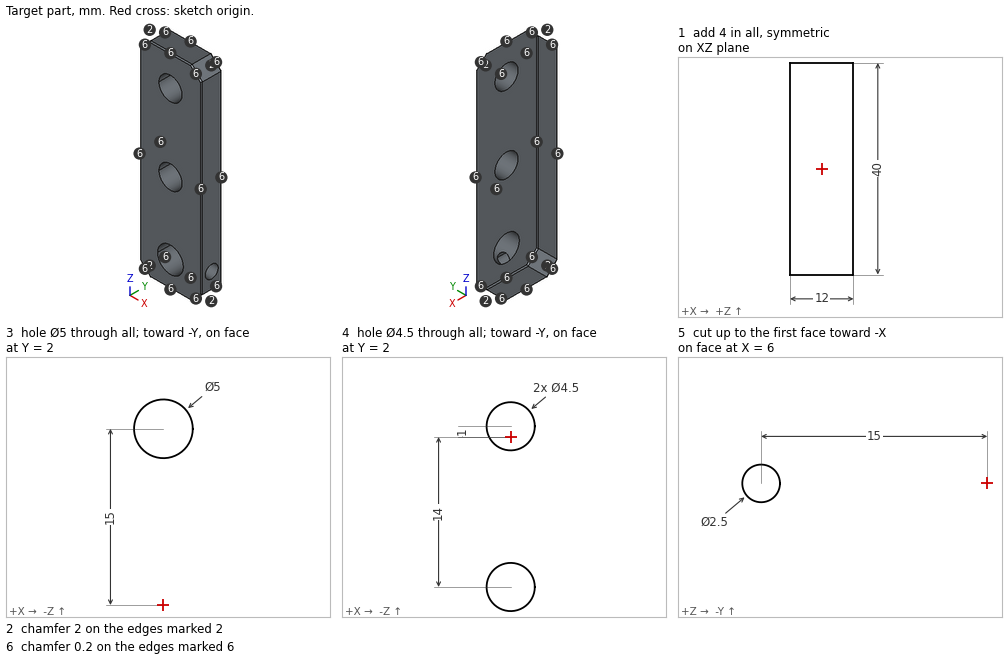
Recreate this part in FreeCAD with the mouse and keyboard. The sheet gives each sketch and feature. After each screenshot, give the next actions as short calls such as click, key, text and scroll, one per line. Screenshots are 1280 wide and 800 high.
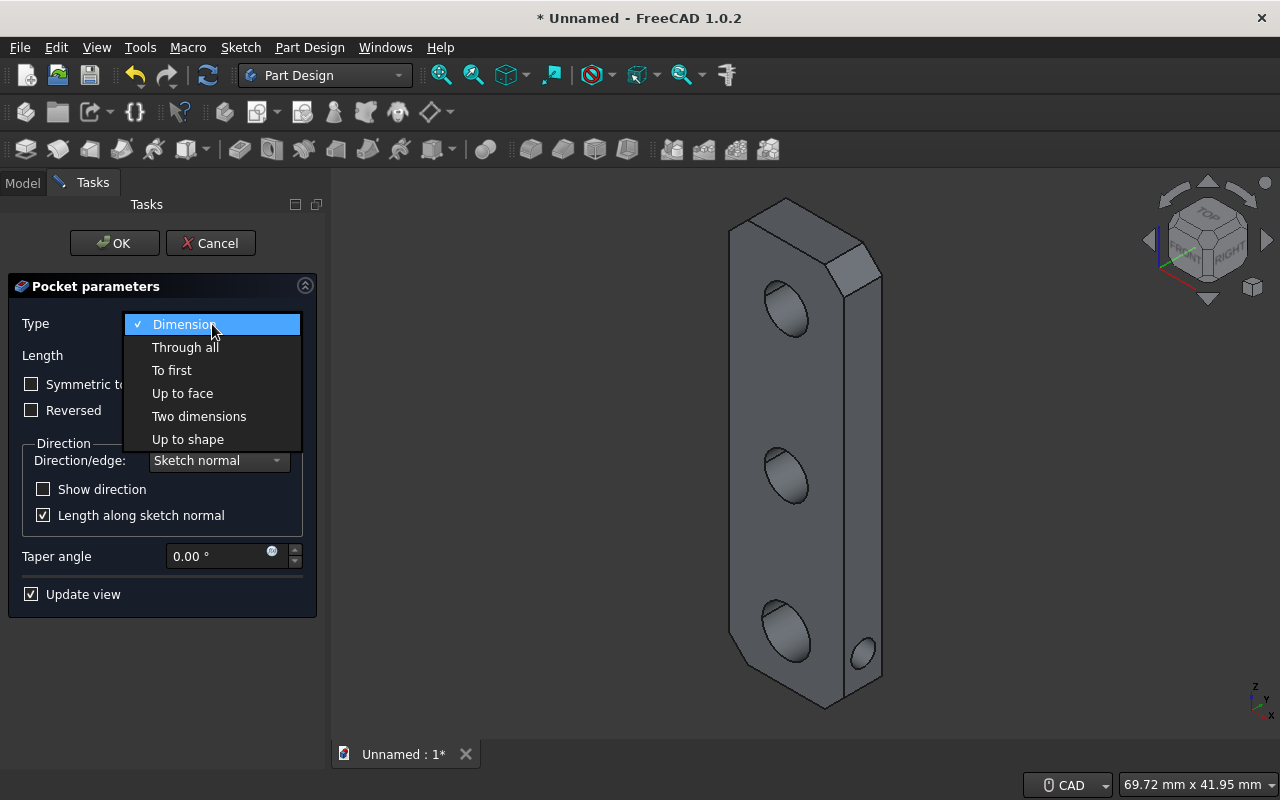
click(212, 370)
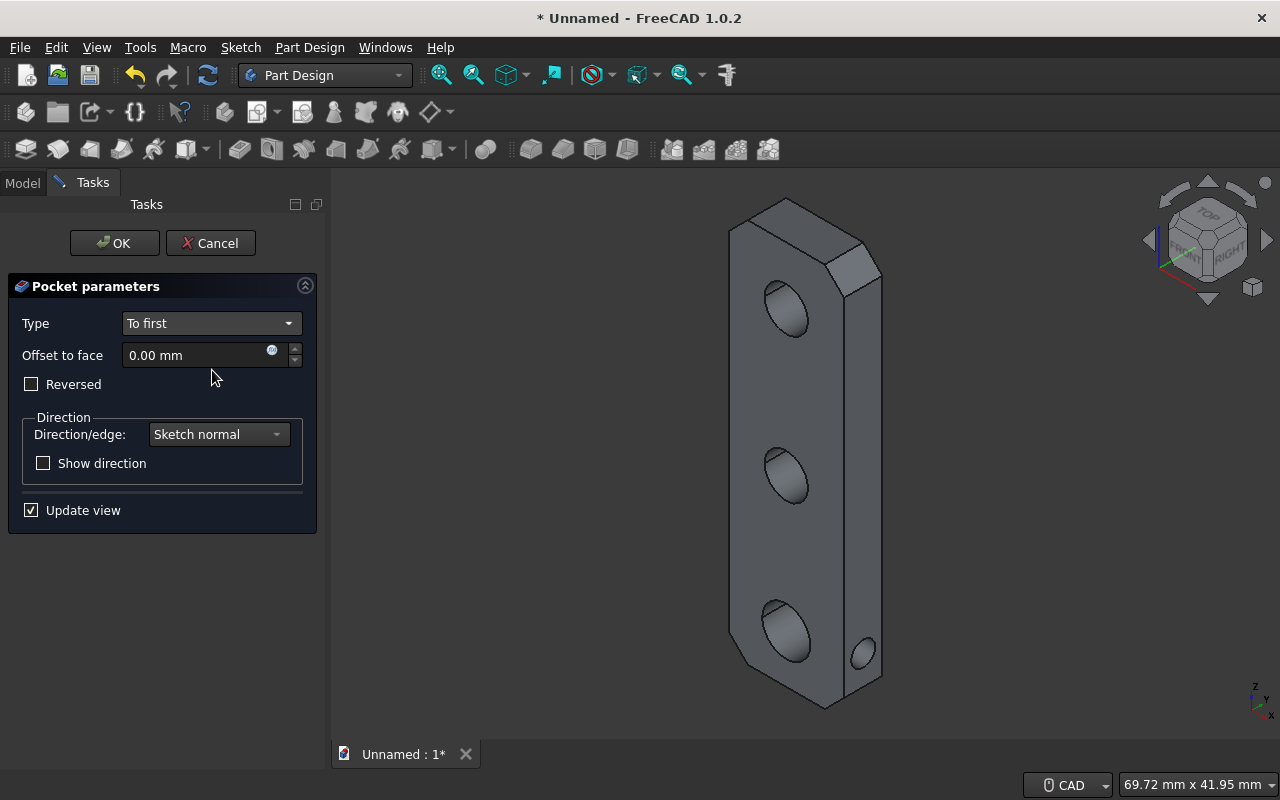
click(115, 243)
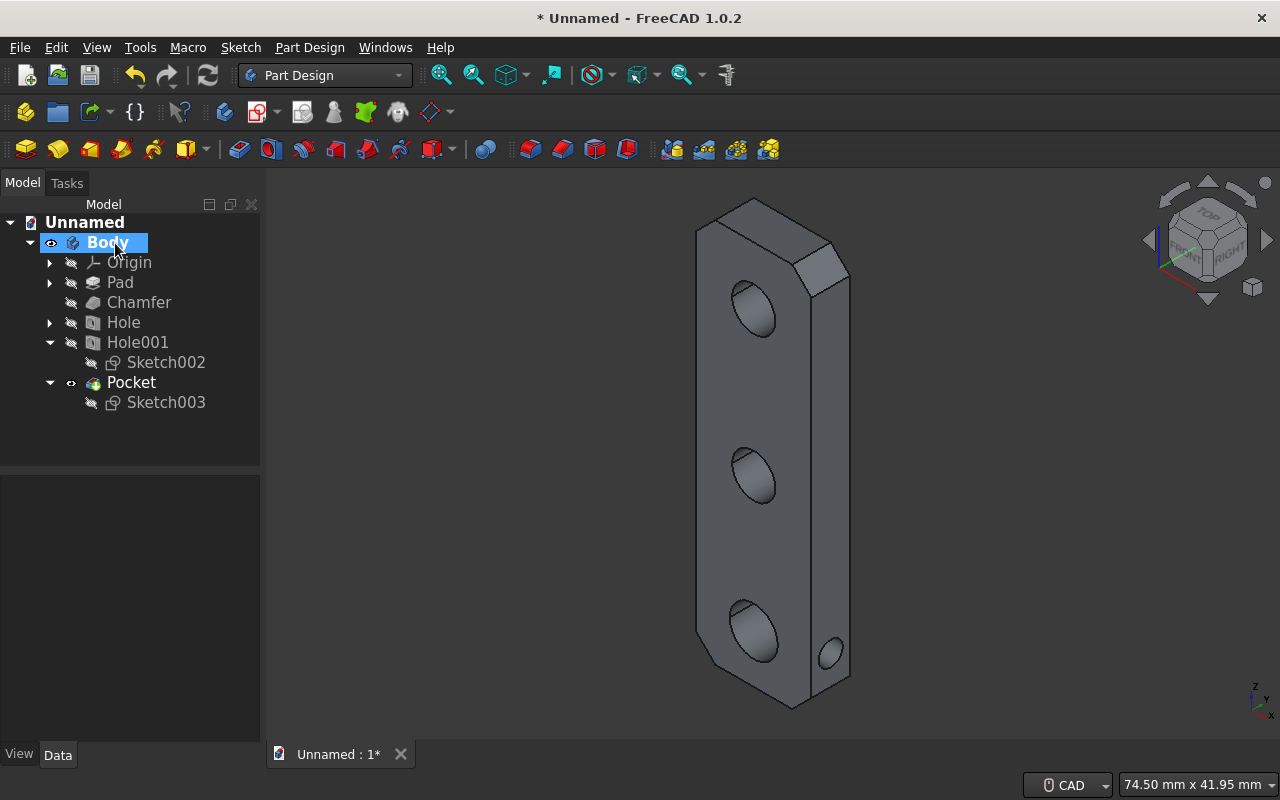
click(811, 497)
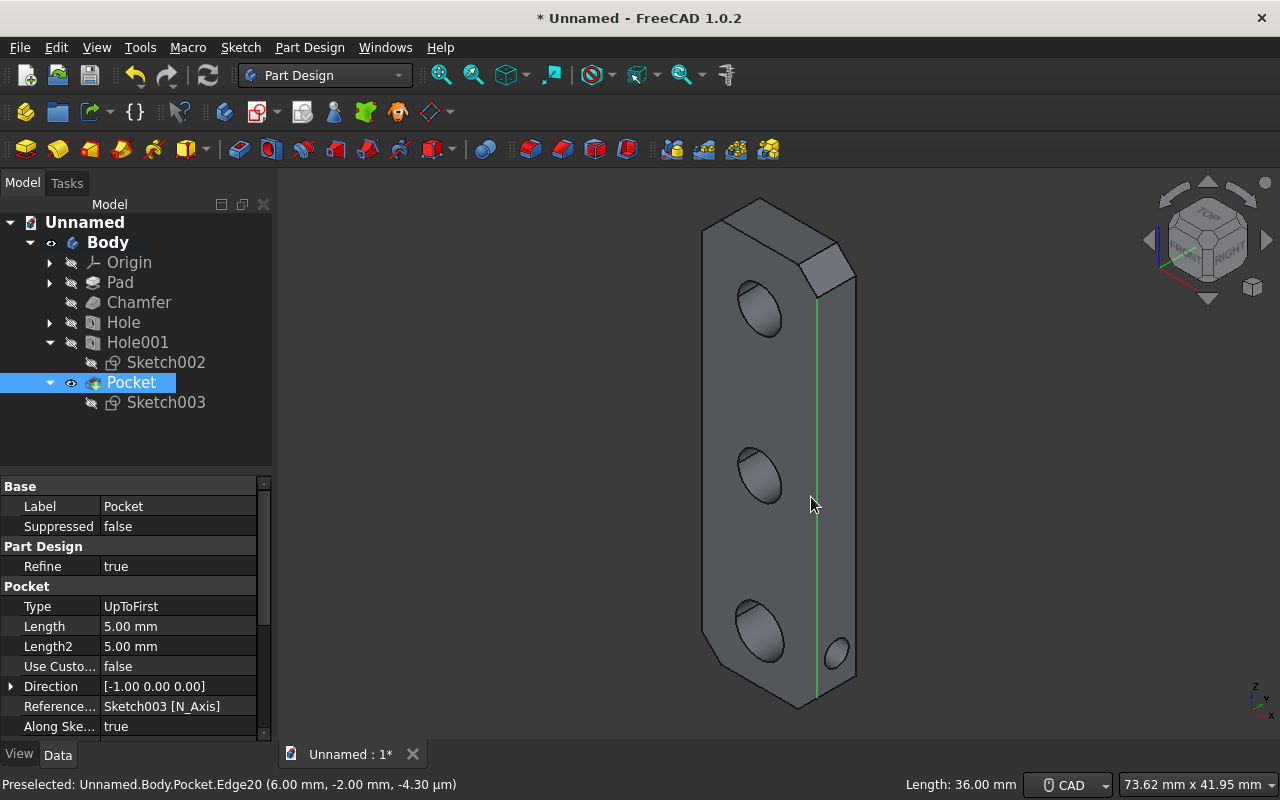
click(760, 241, ctrl)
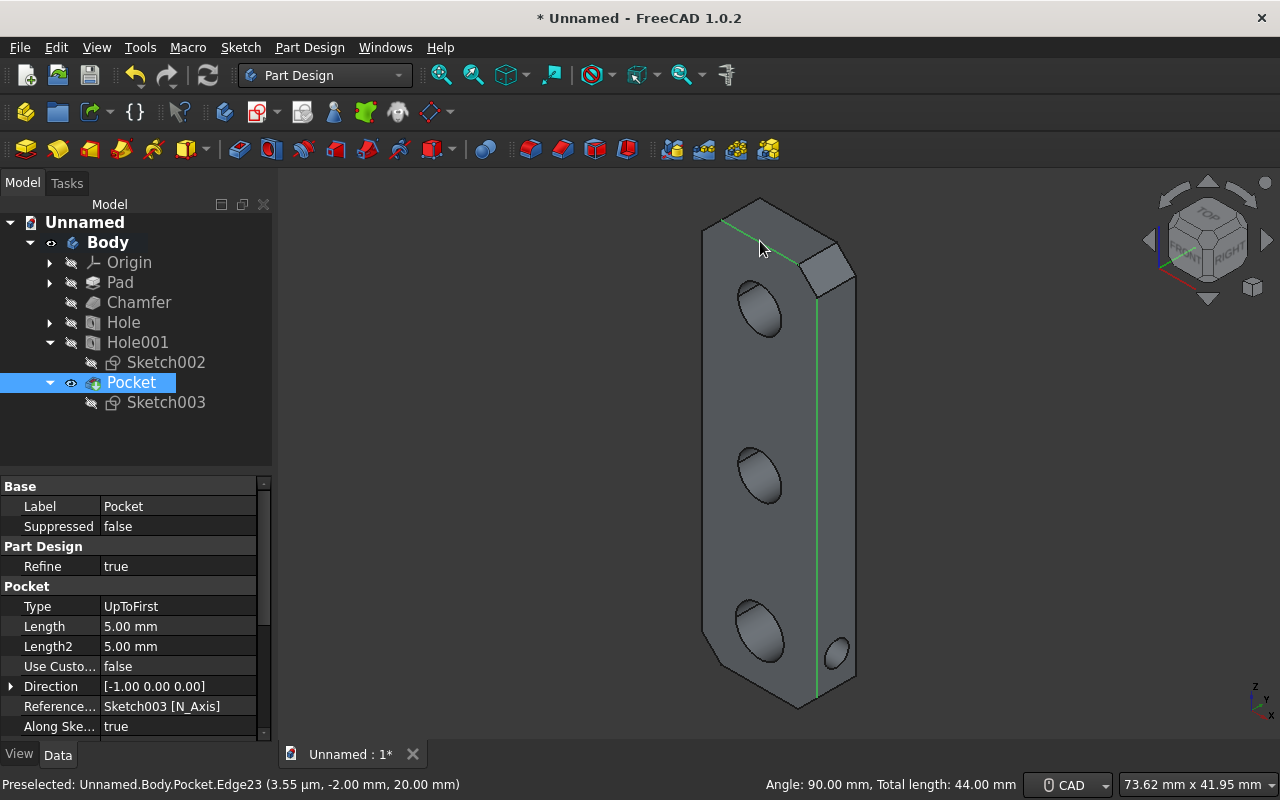
click(712, 225, ctrl)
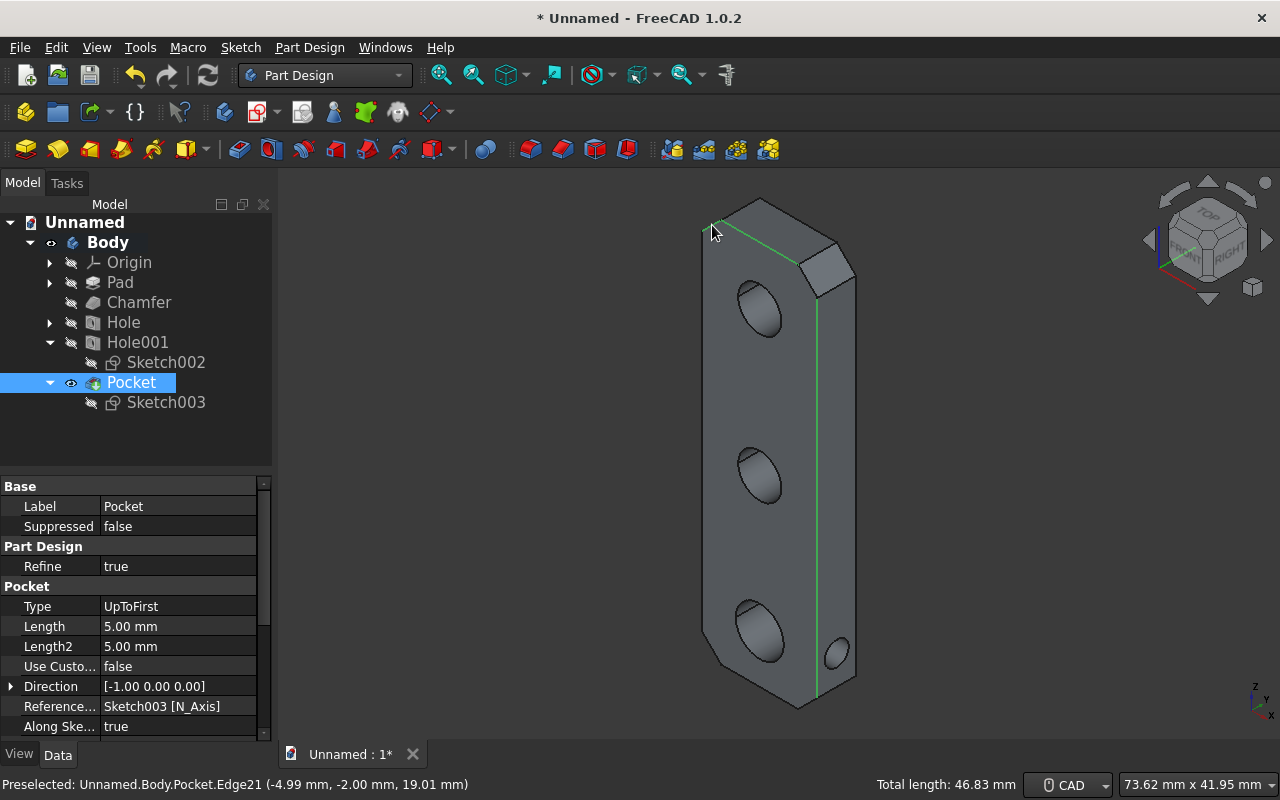
click(808, 280, ctrl)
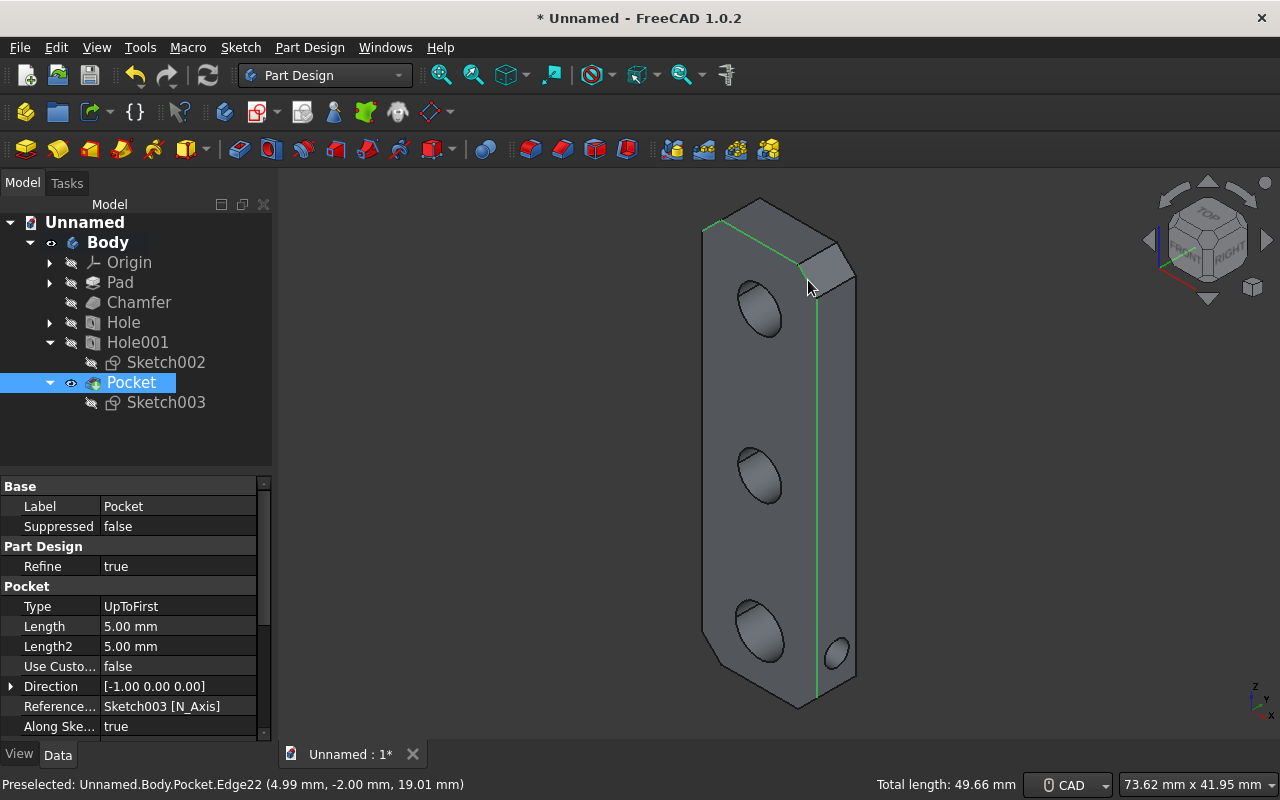
click(808, 703, ctrl)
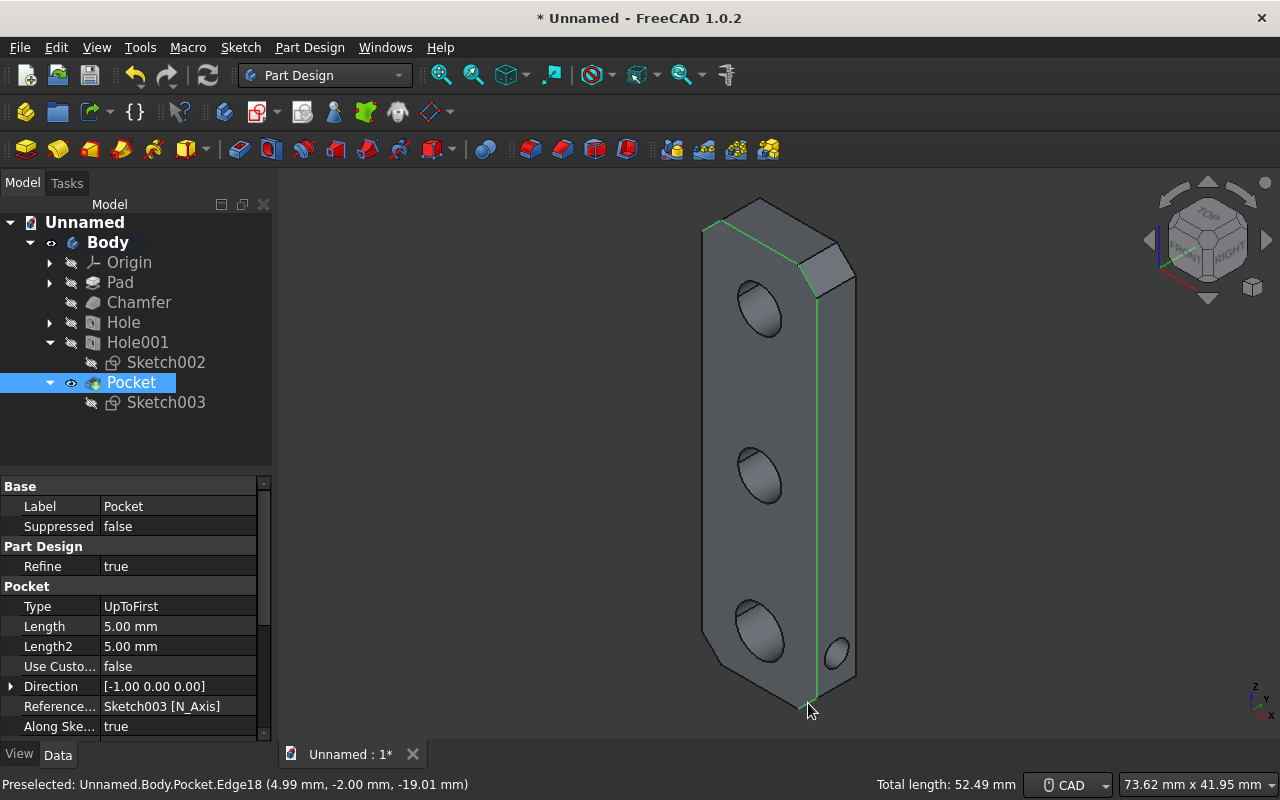
key(2)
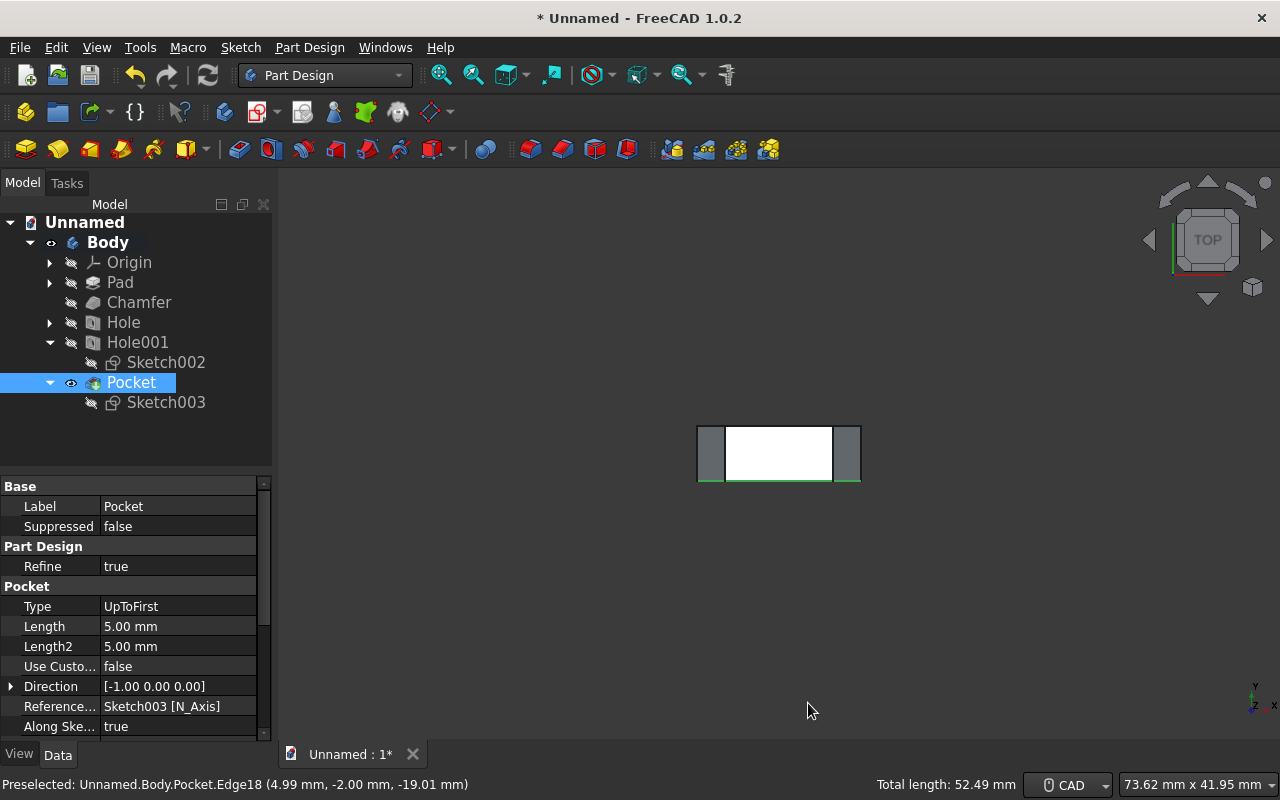
click(442, 76)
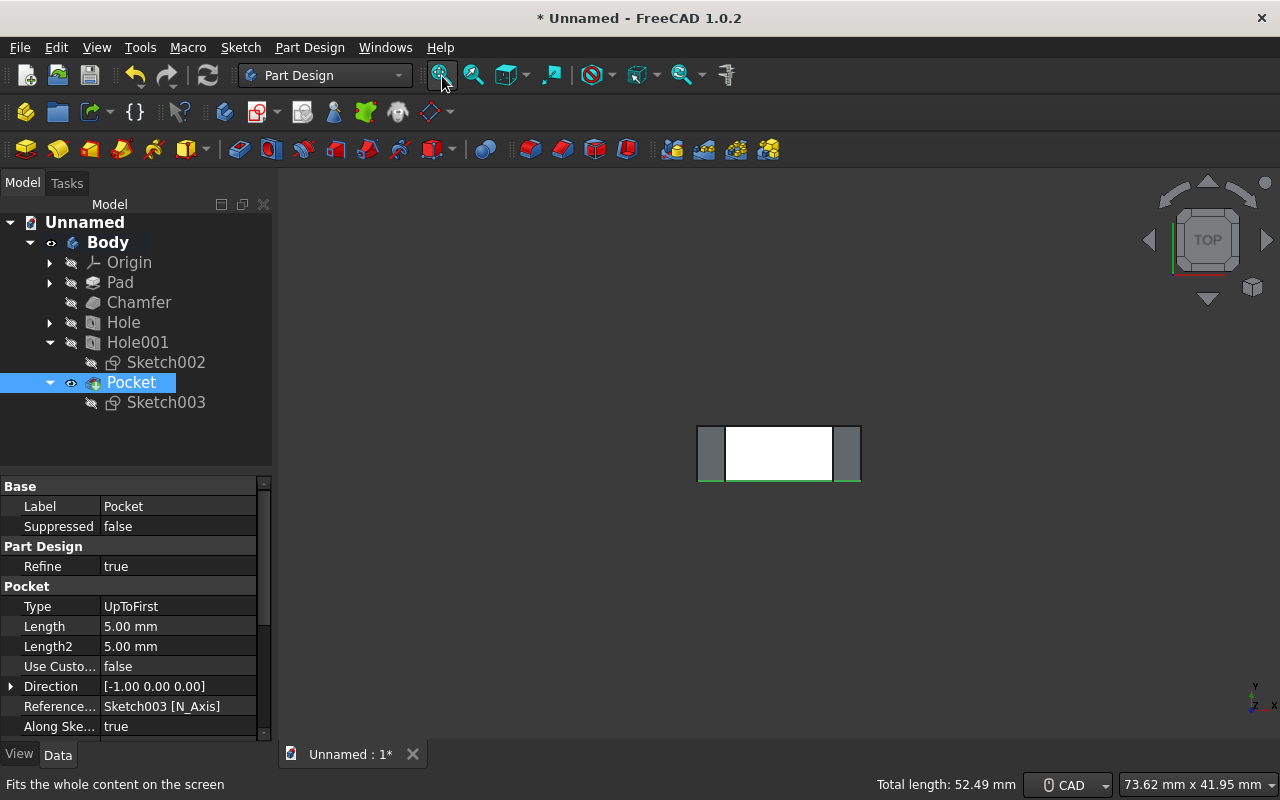
click(779, 425, ctrl)